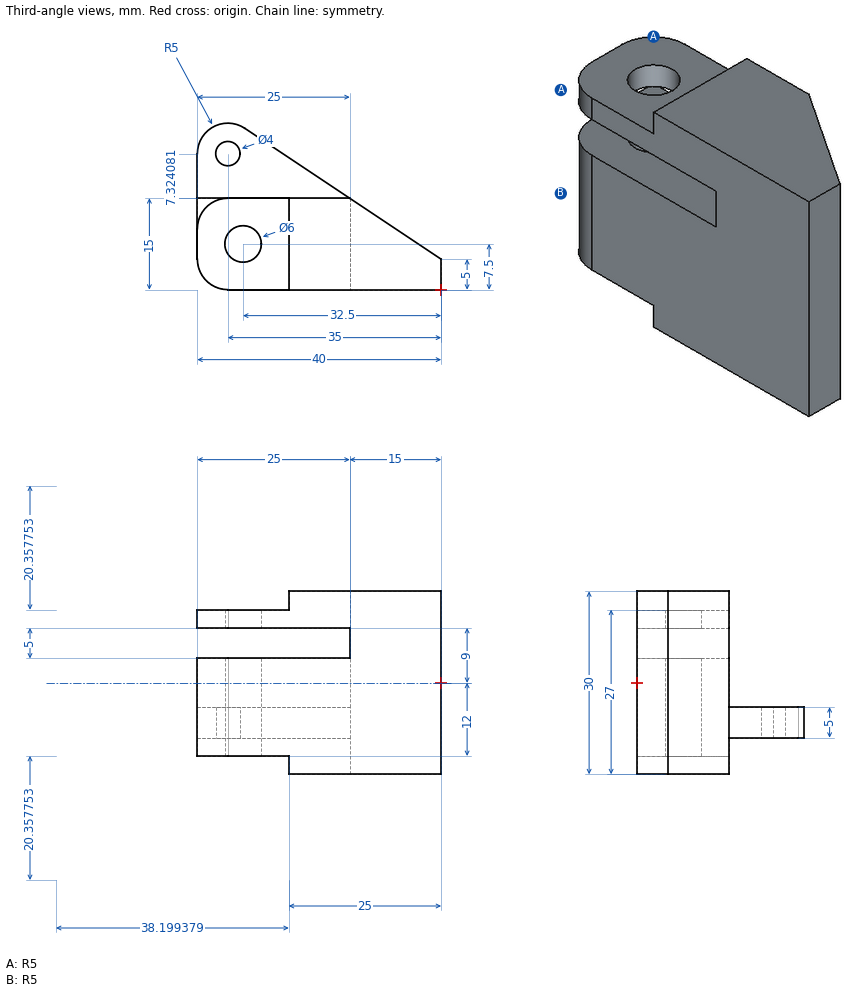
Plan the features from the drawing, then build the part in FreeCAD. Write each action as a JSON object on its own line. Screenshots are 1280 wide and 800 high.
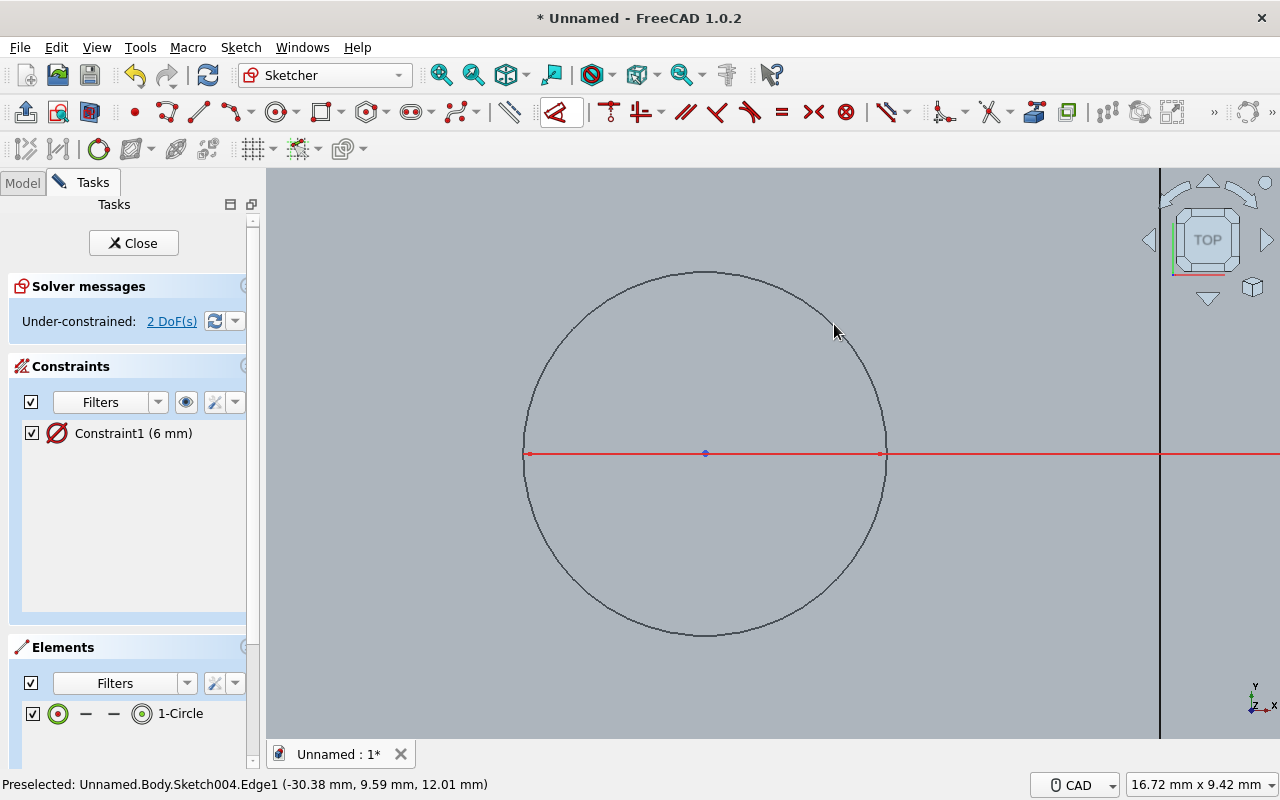
{"action": "left_click", "coordinate": [705, 454]}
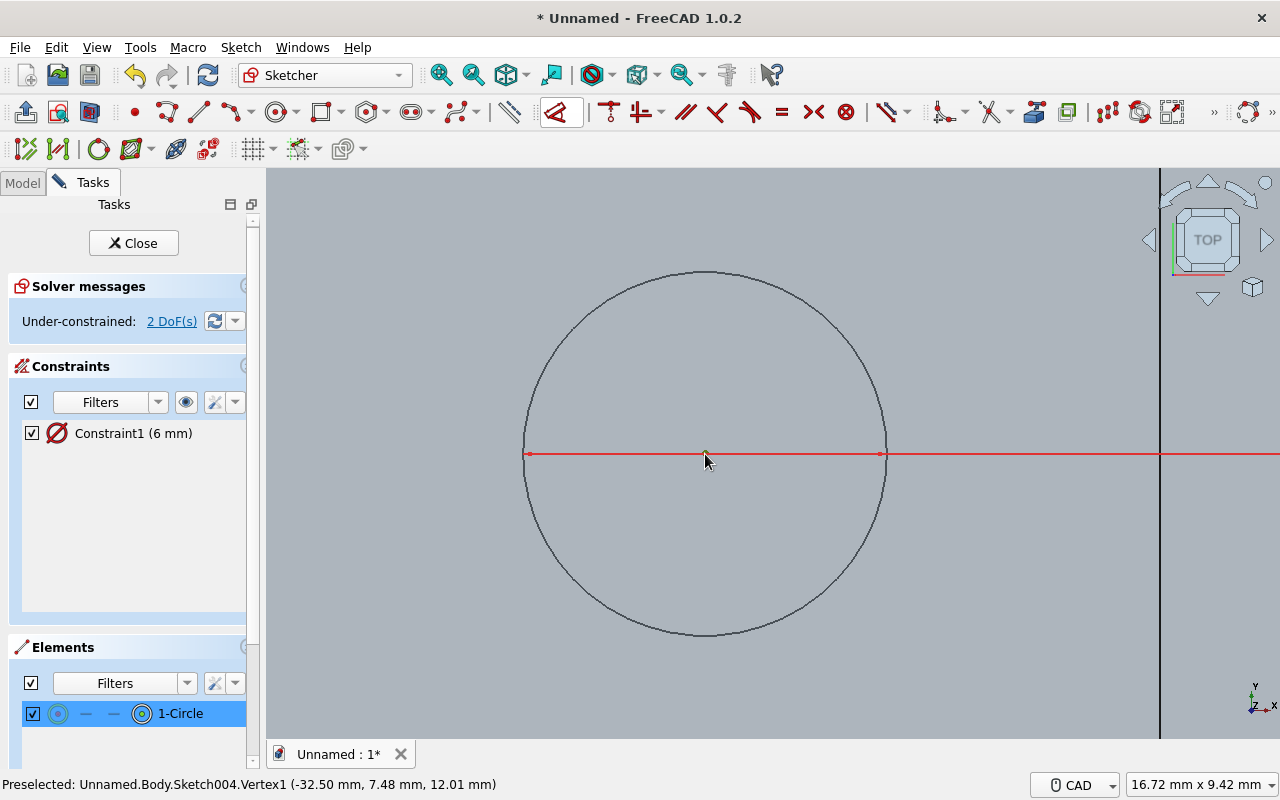
{"action": "key", "text": "i"}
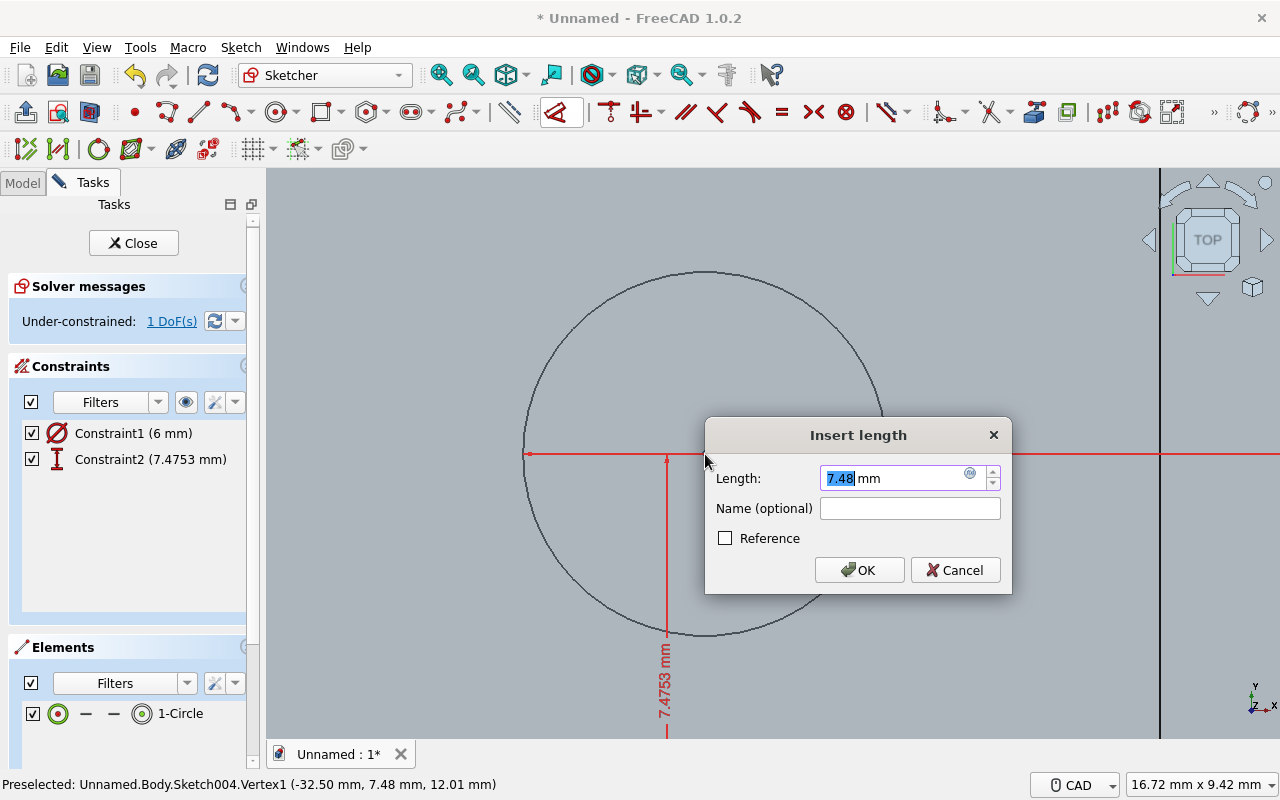
{"action": "type", "text": "7.5"}
{"action": "key", "text": "Return"}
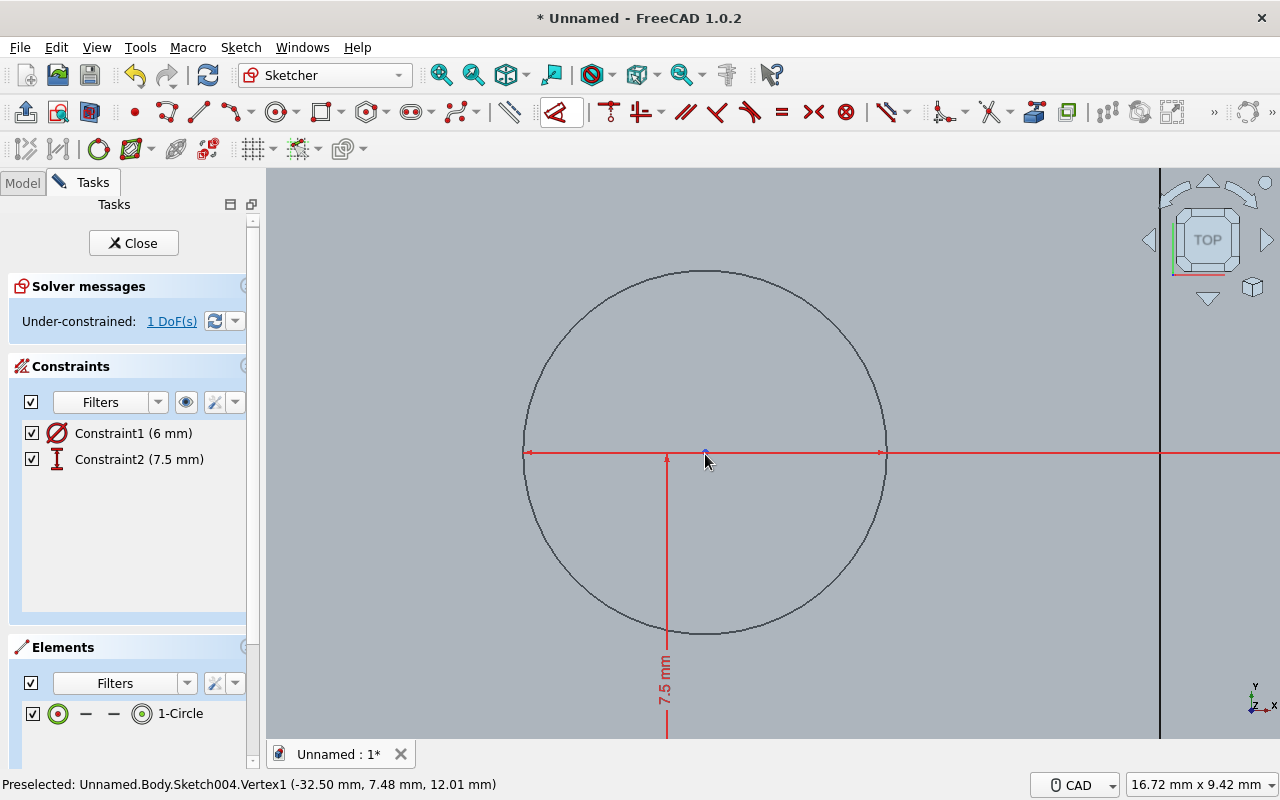
{"action": "left_click", "coordinate": [705, 453]}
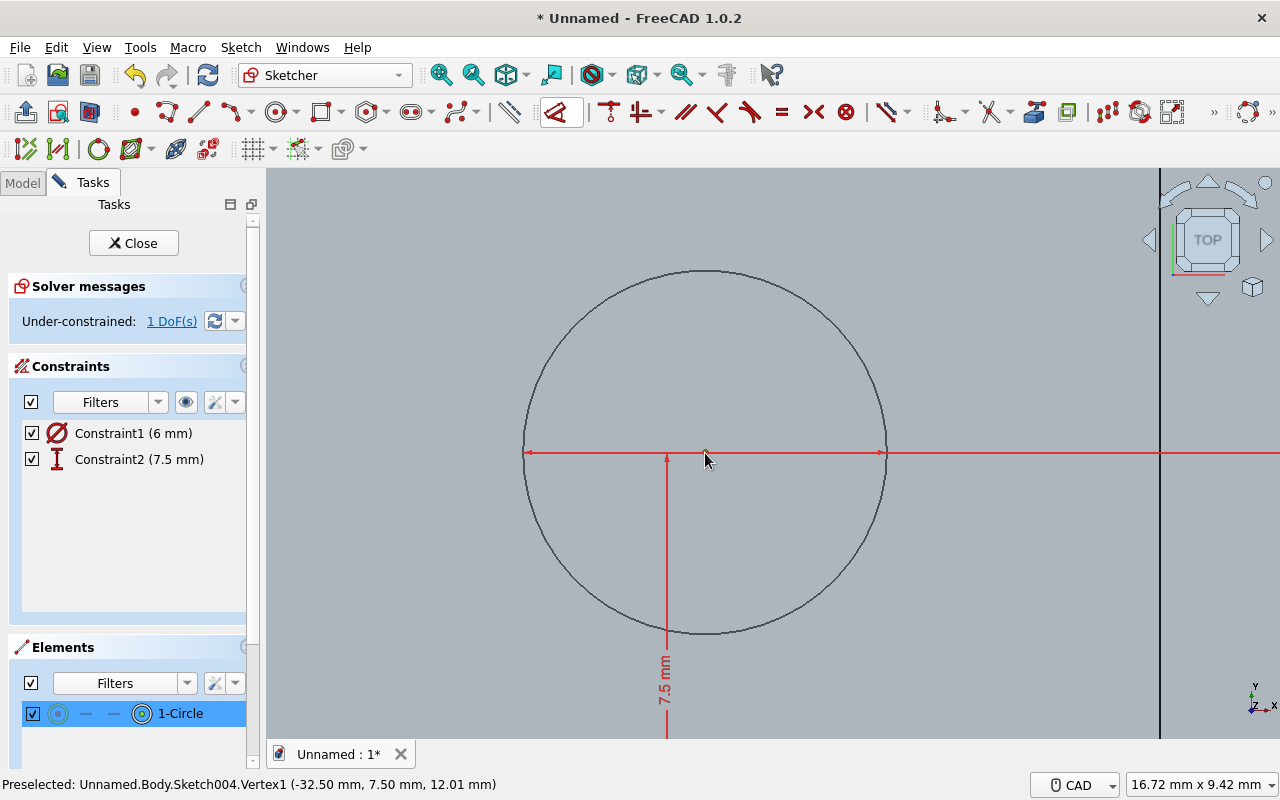
{"action": "key", "text": "l"}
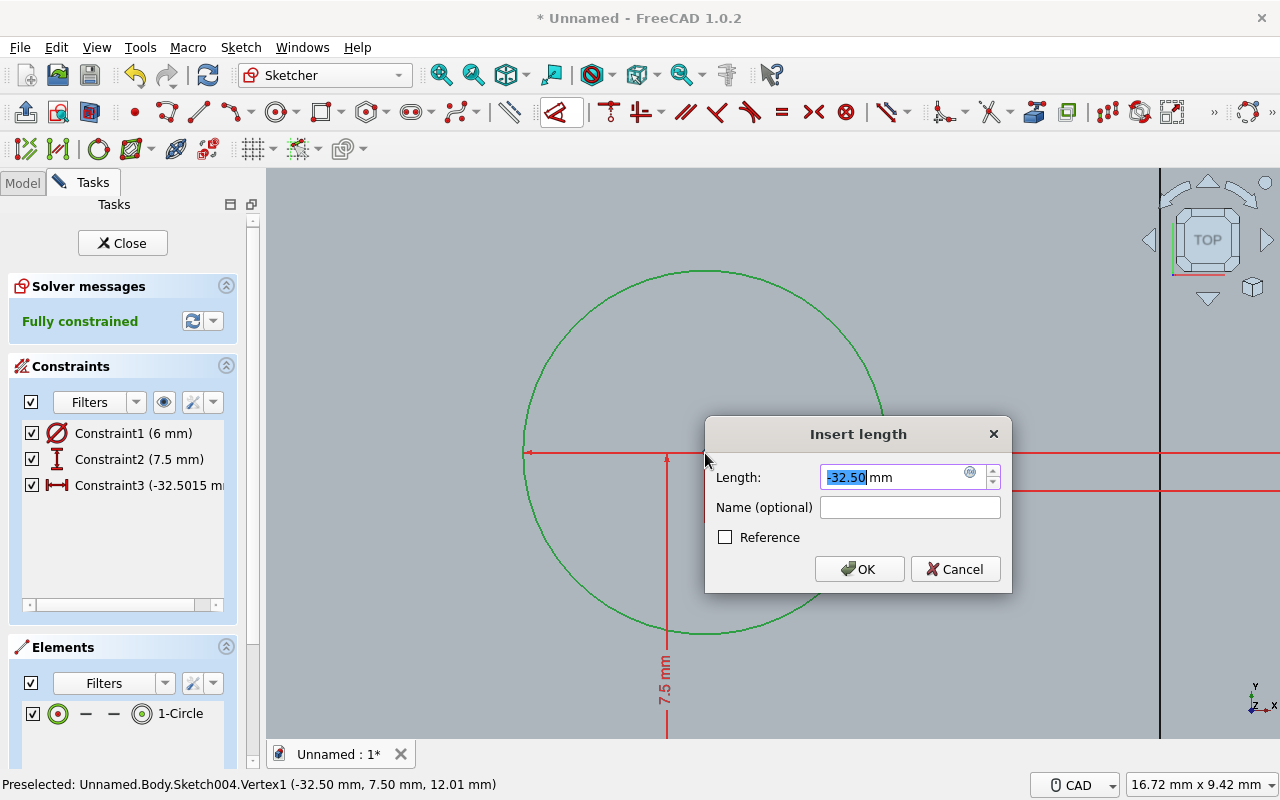
{"action": "type", "text": "-32.5"}
{"action": "key", "text": "Return"}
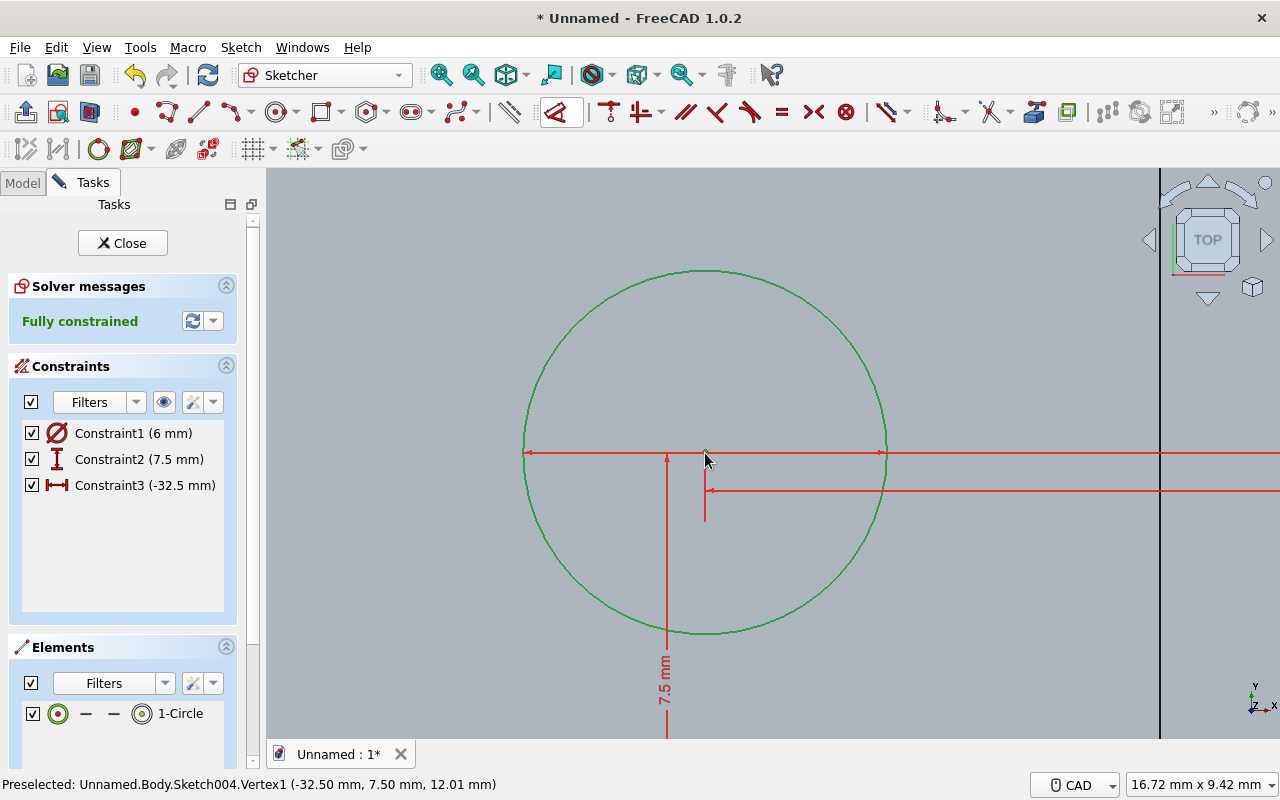
{"action": "left_click", "coordinate": [123, 243]}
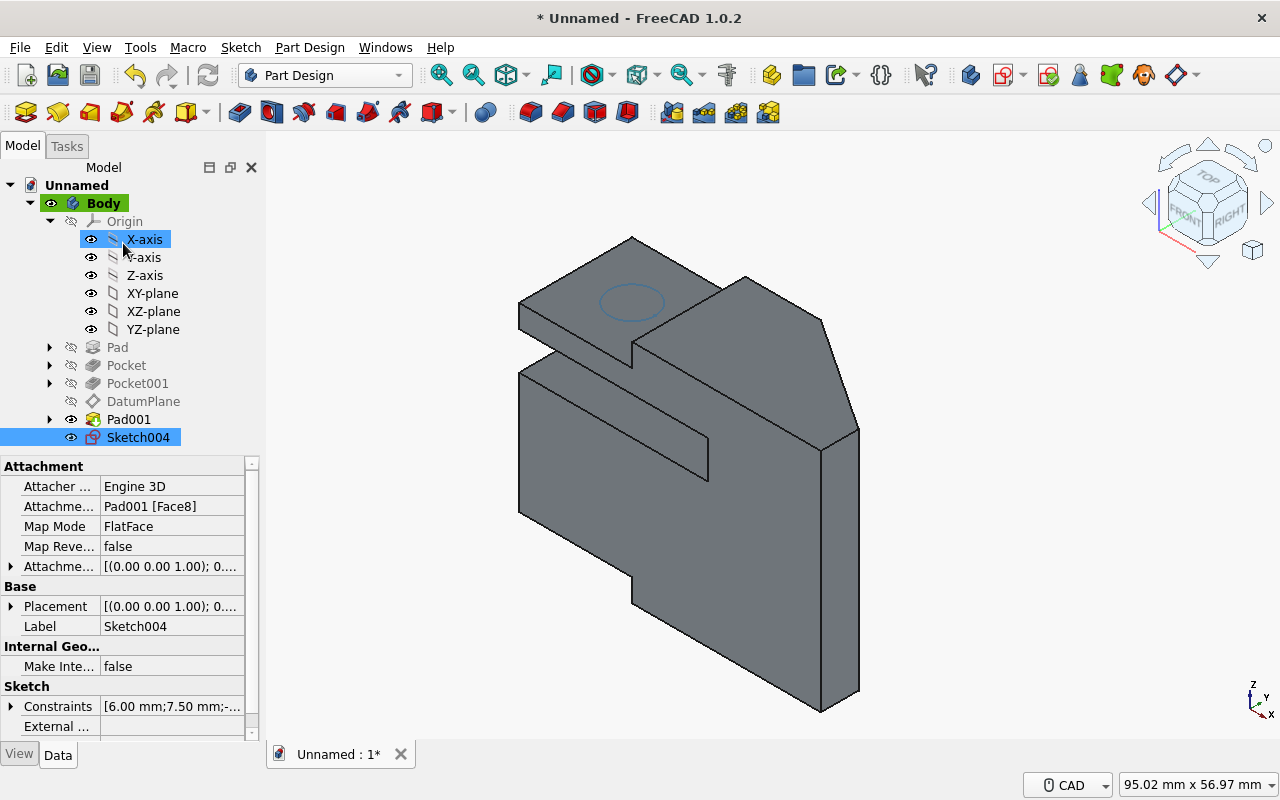
{"action": "left_click", "coordinate": [240, 112]}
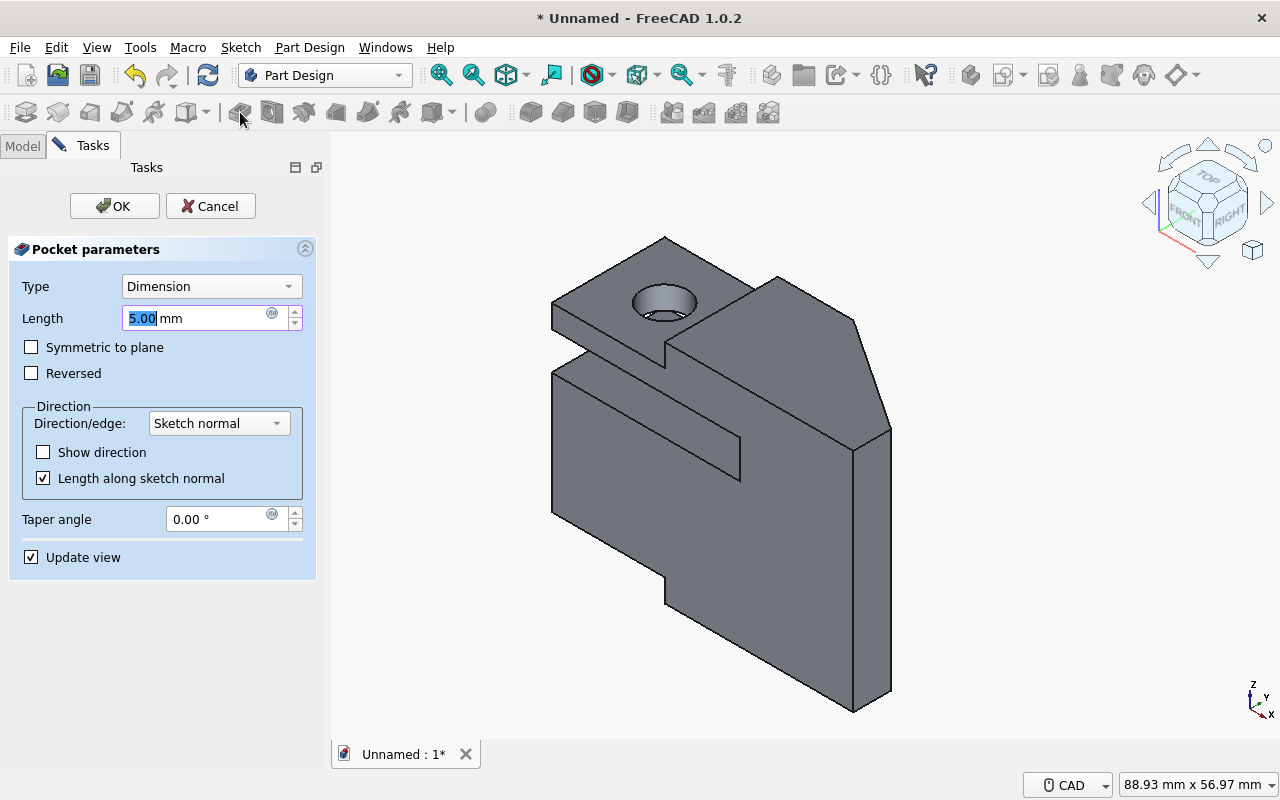
{"action": "type", "text": "27"}
{"action": "key", "text": "Tab"}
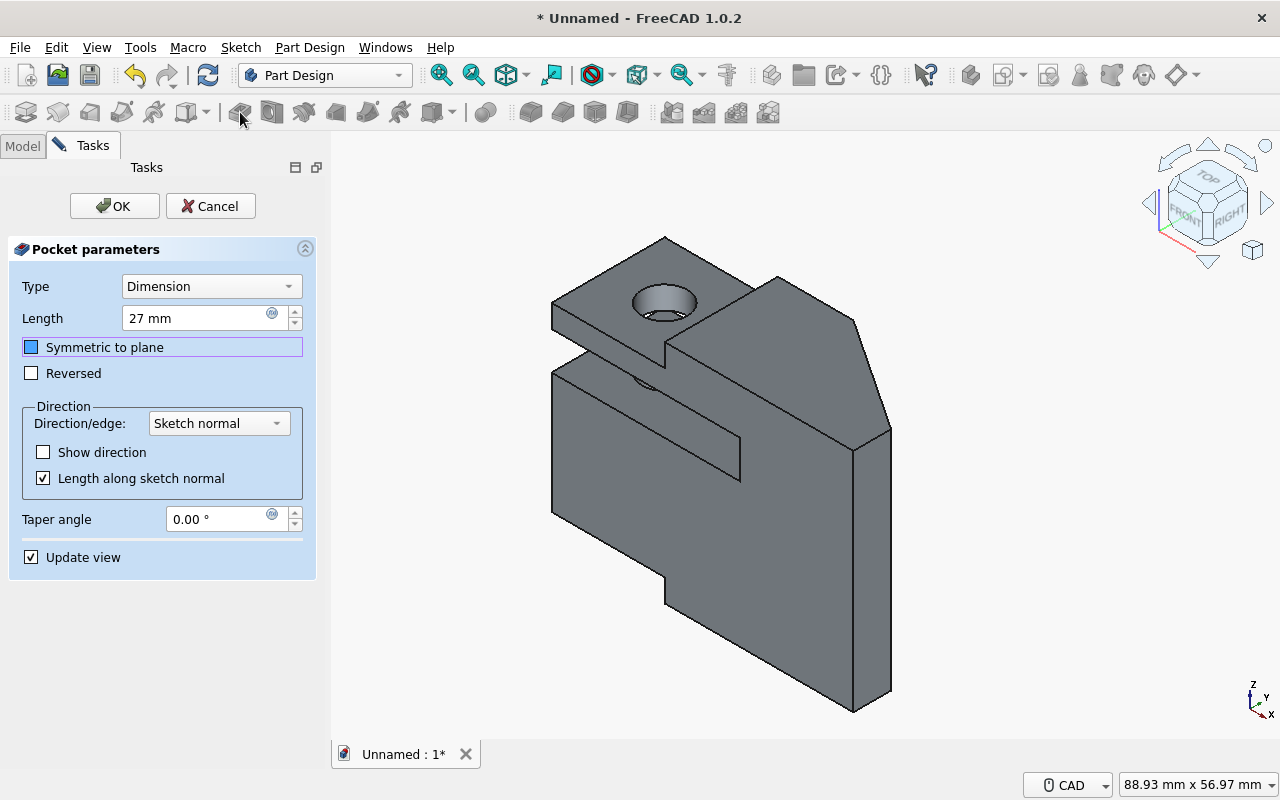
{"action": "left_click", "coordinate": [115, 206]}